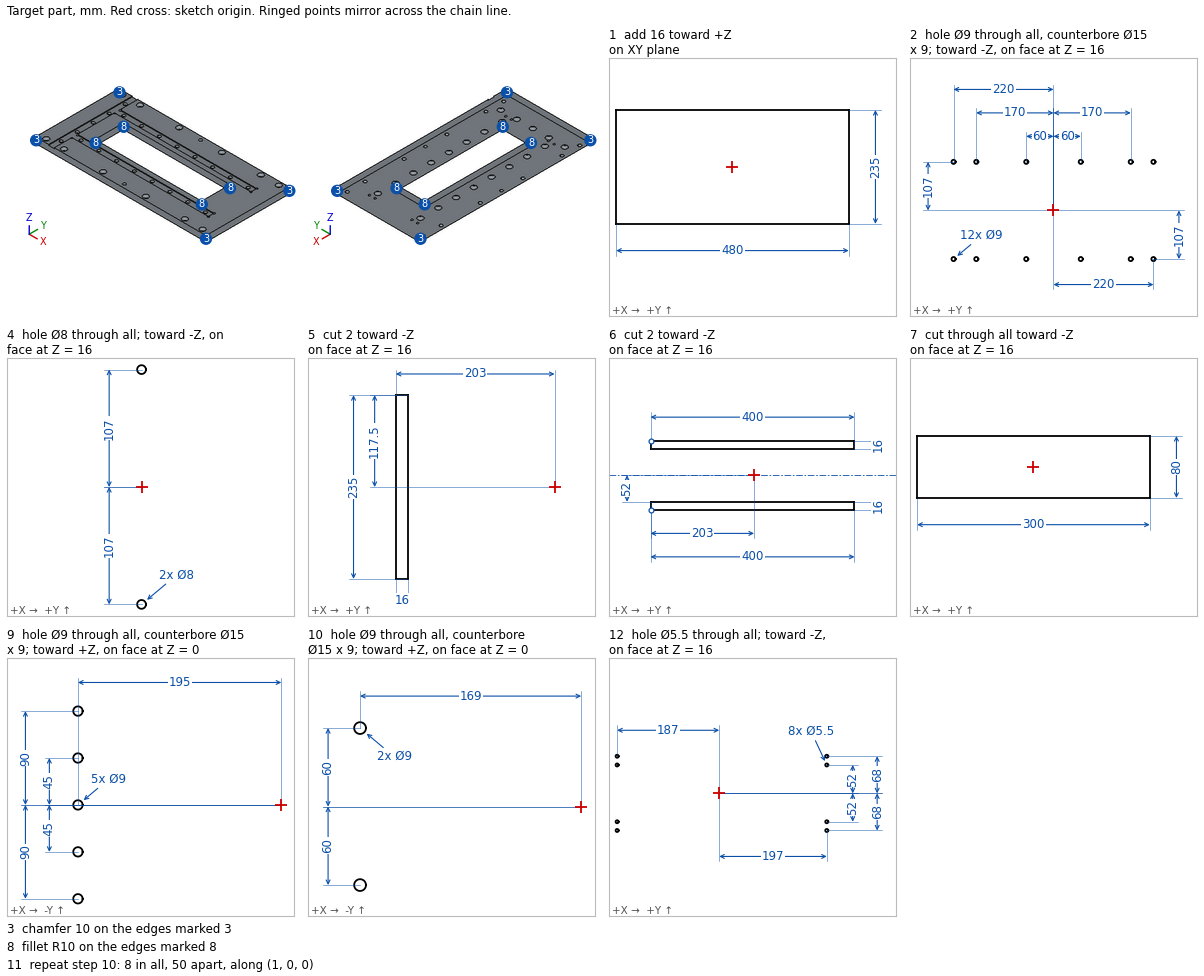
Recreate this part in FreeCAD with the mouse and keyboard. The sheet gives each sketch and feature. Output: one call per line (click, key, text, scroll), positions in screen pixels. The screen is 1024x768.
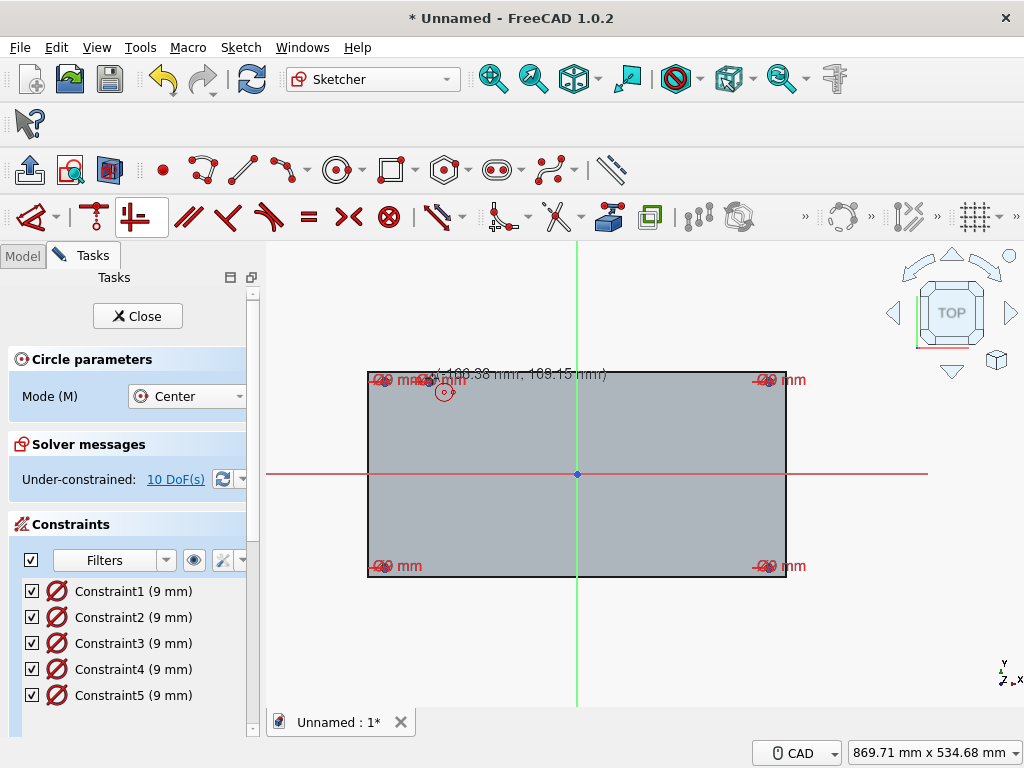
scroll(429, 567, up, 9)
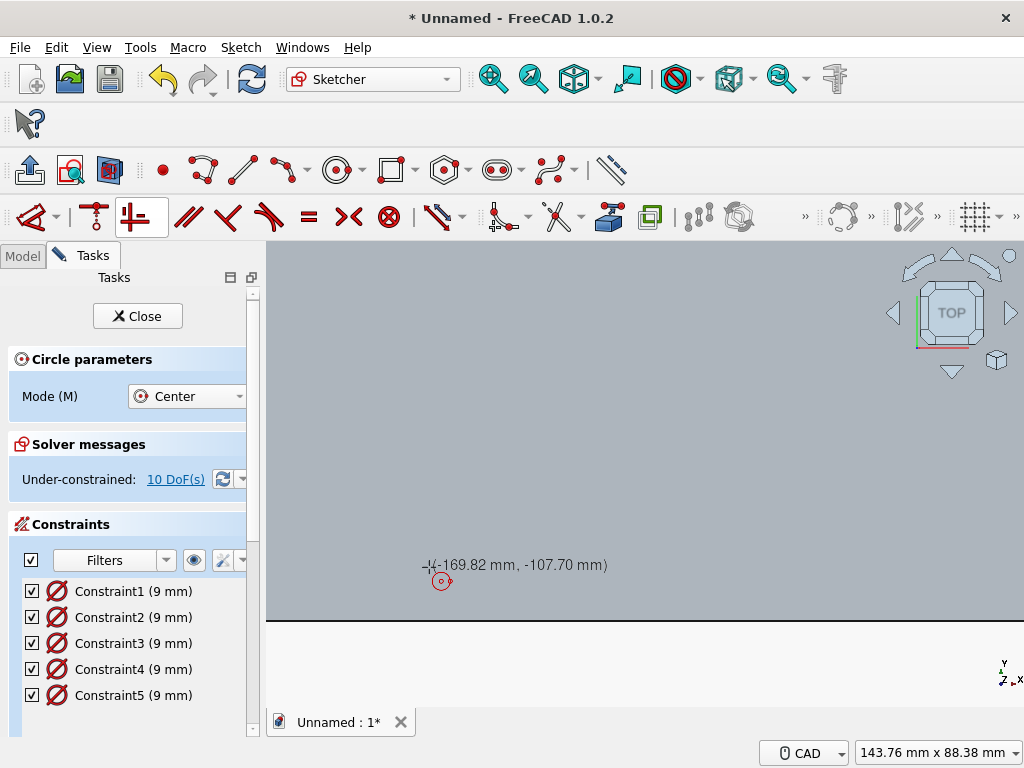
scroll(429, 568, down, 9)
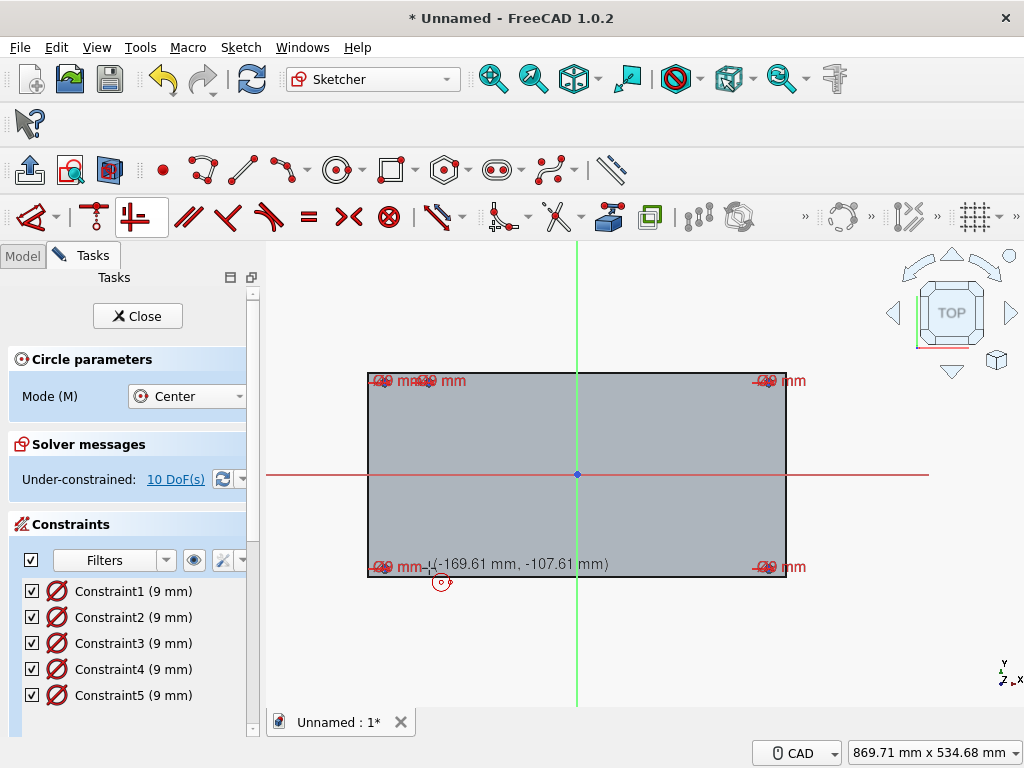
click(429, 568)
move(432, 565)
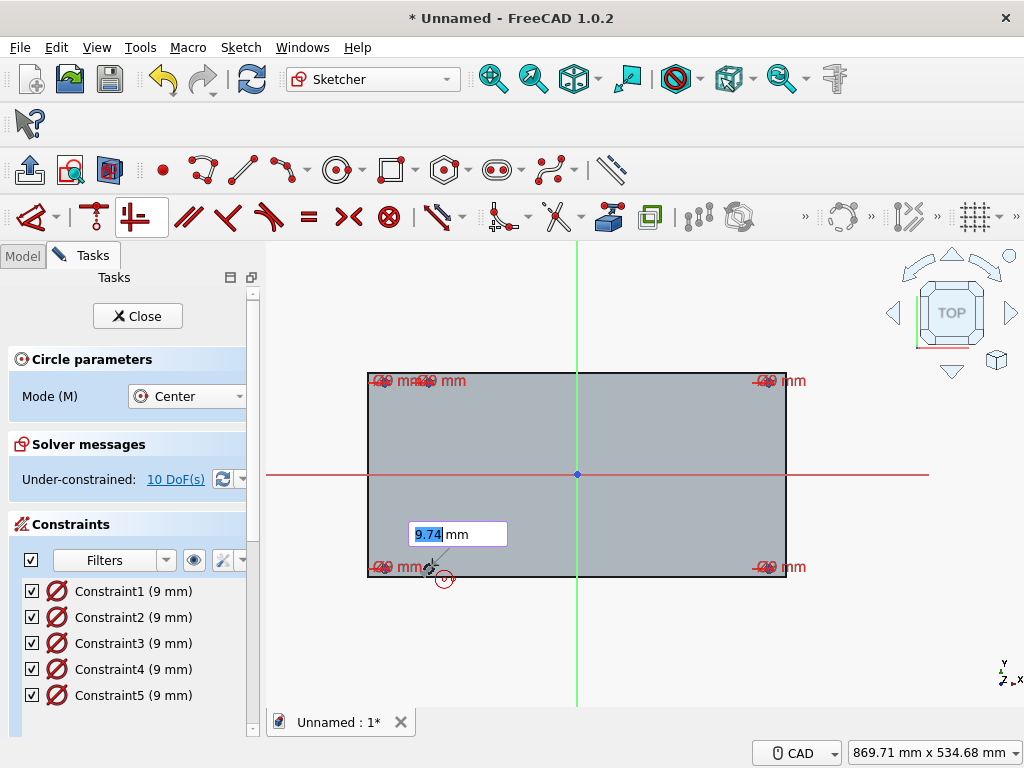
text(9)
key(Return)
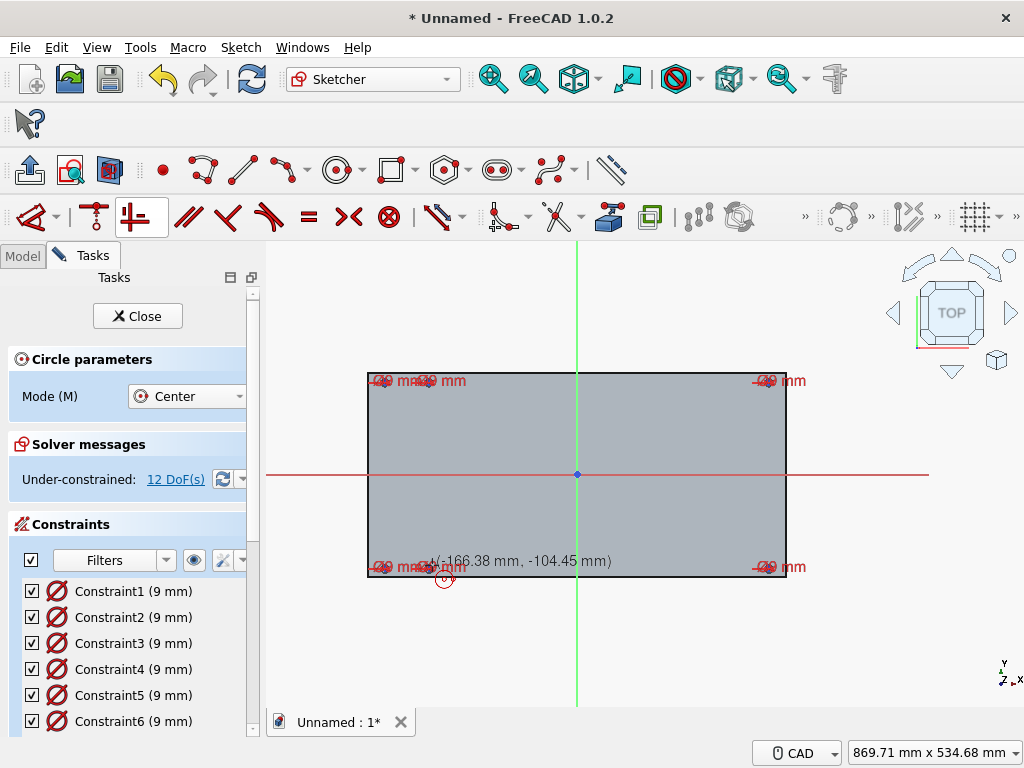
scroll(525, 382, up, 9)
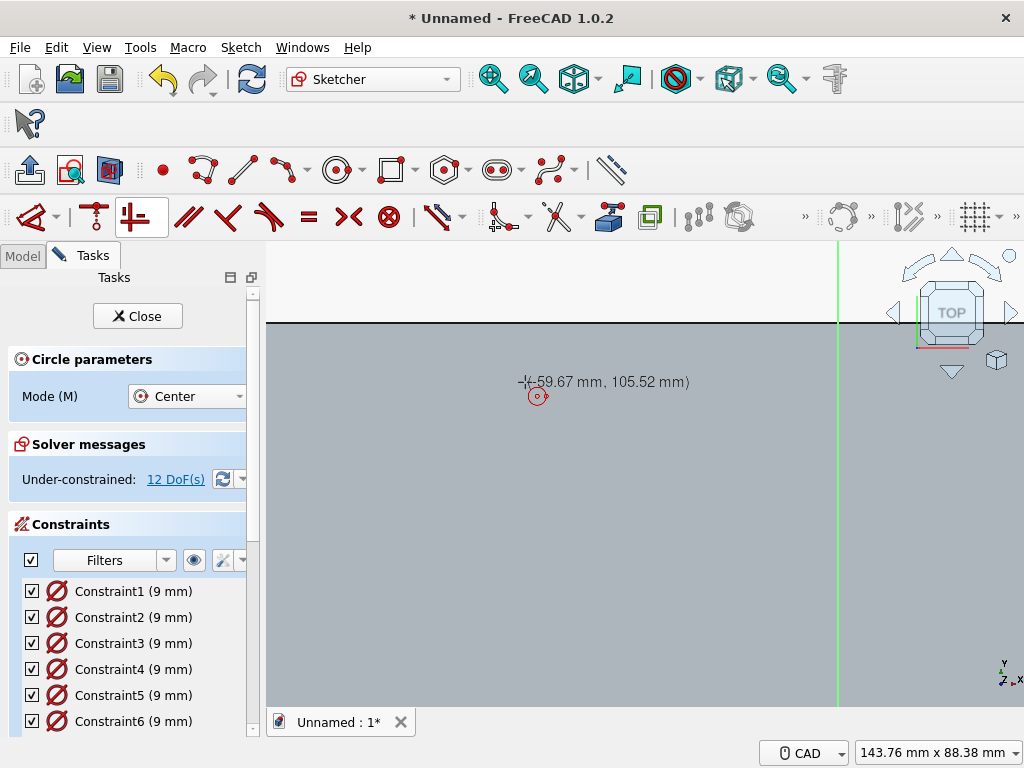
scroll(525, 381, down, 9)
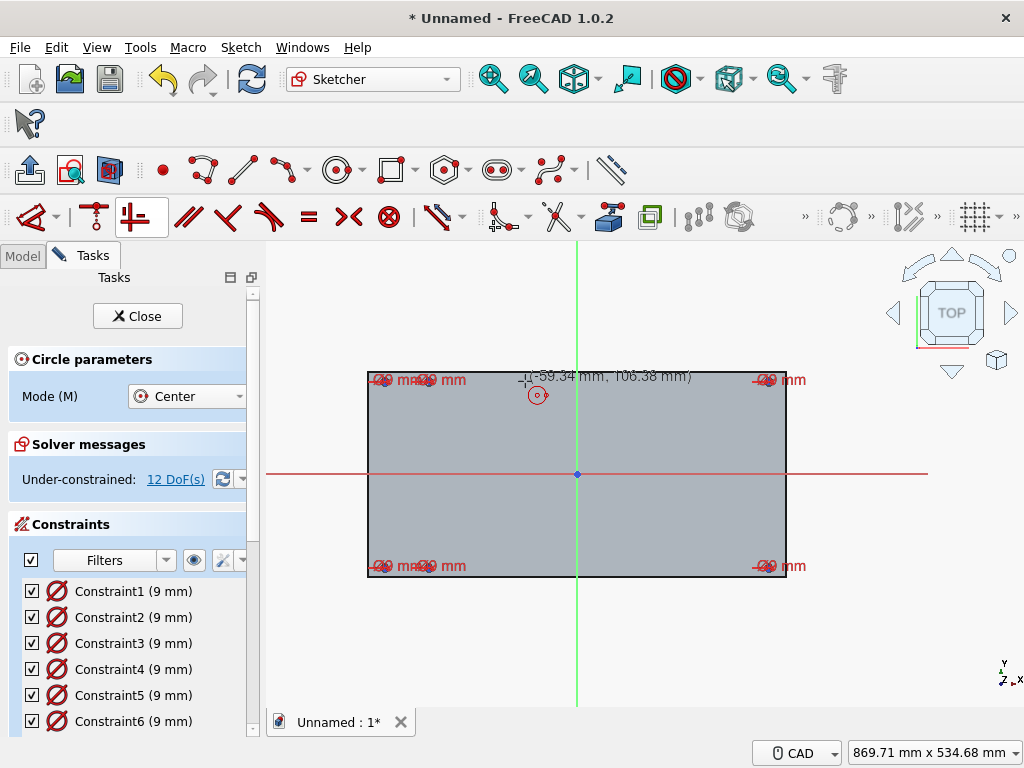
click(525, 381)
move(527, 378)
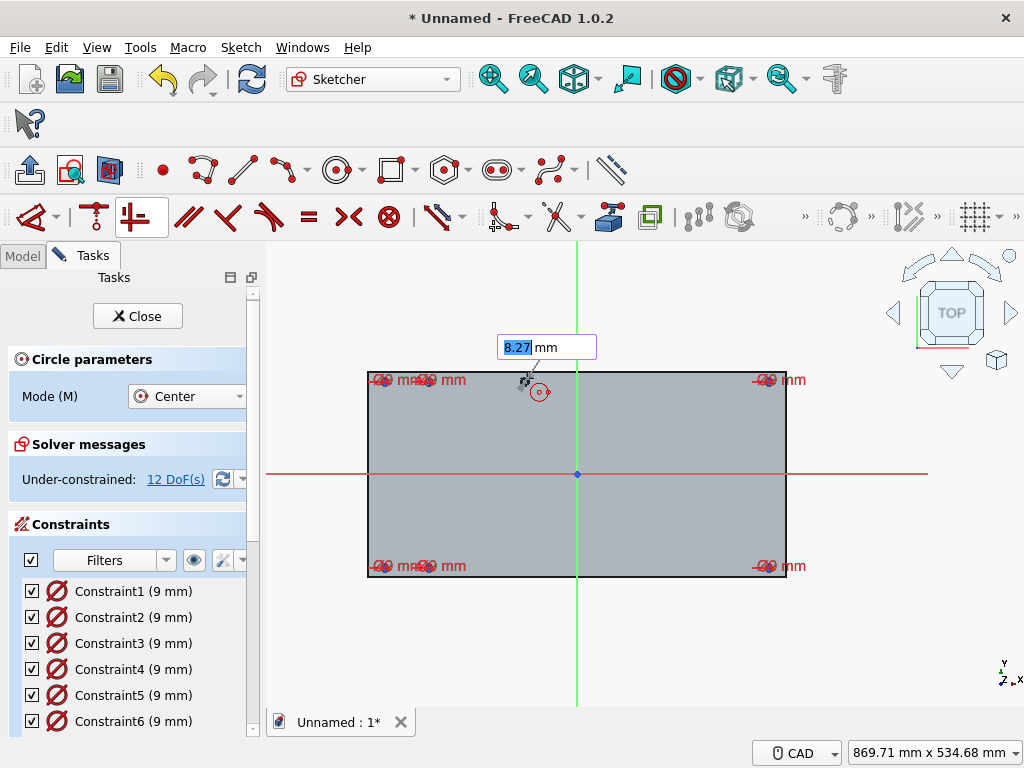
text(9)
key(Return)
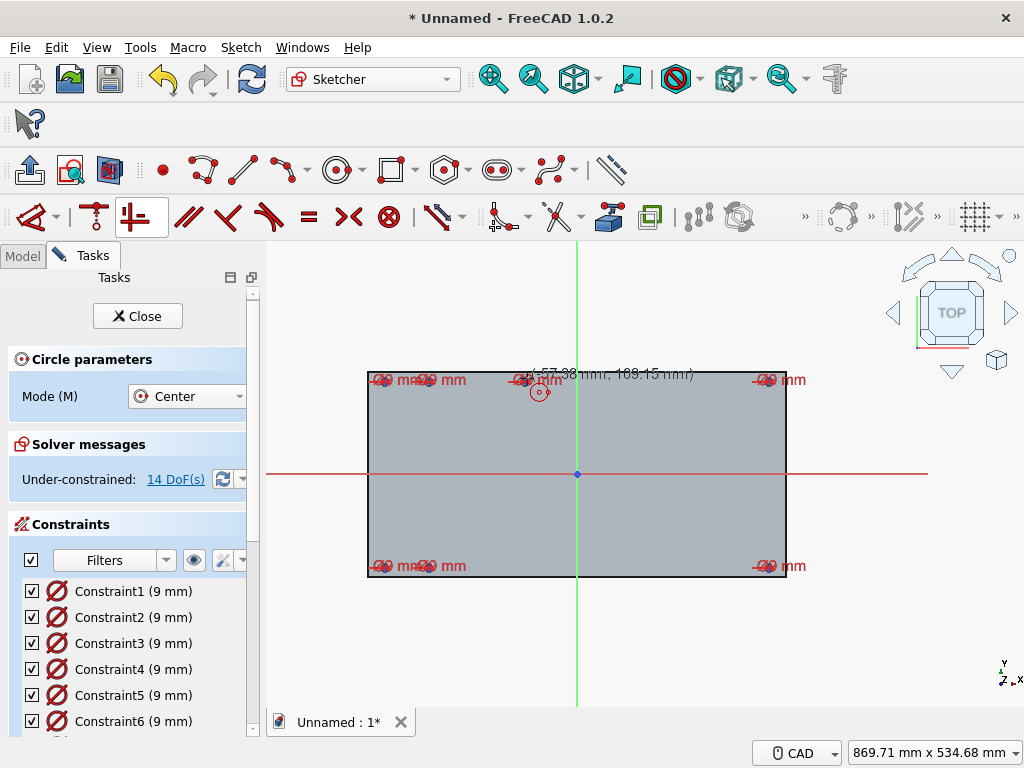
scroll(525, 567, up, 9)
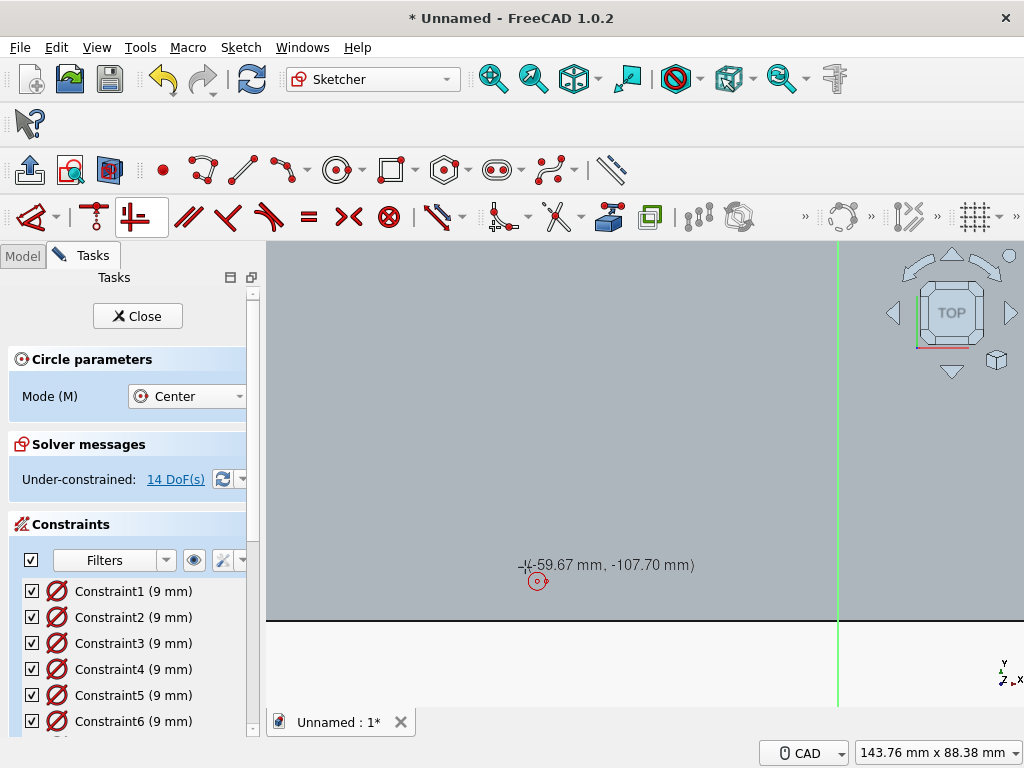
scroll(525, 568, down, 9)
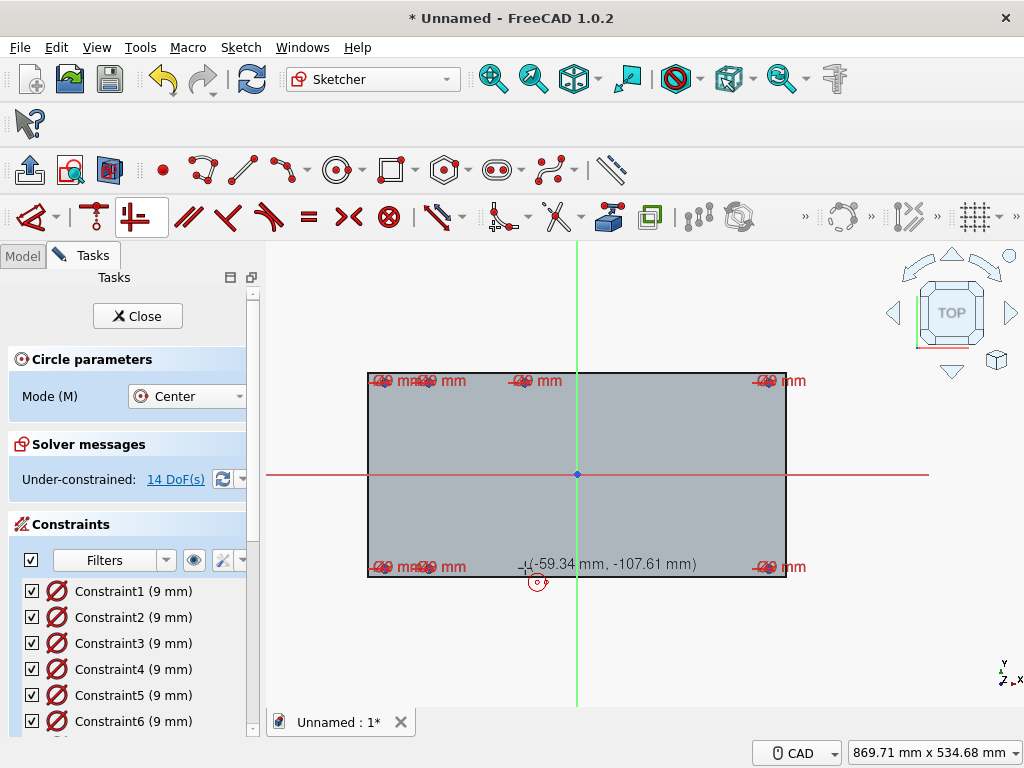
click(525, 568)
move(527, 565)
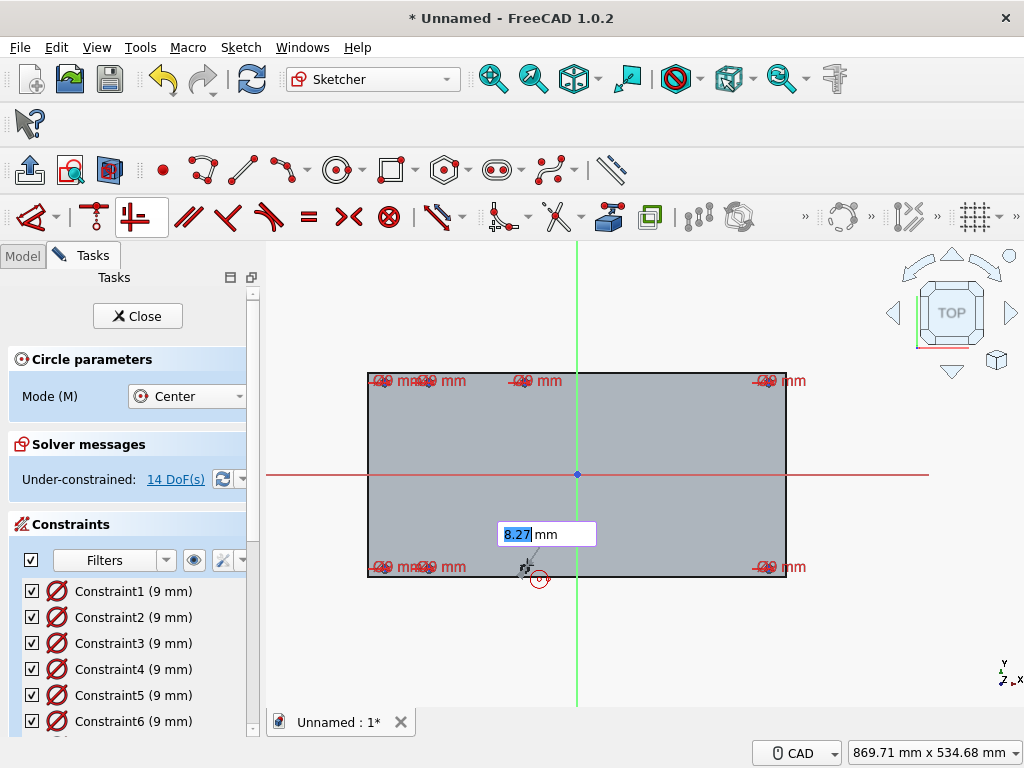
text(9)
key(Return)